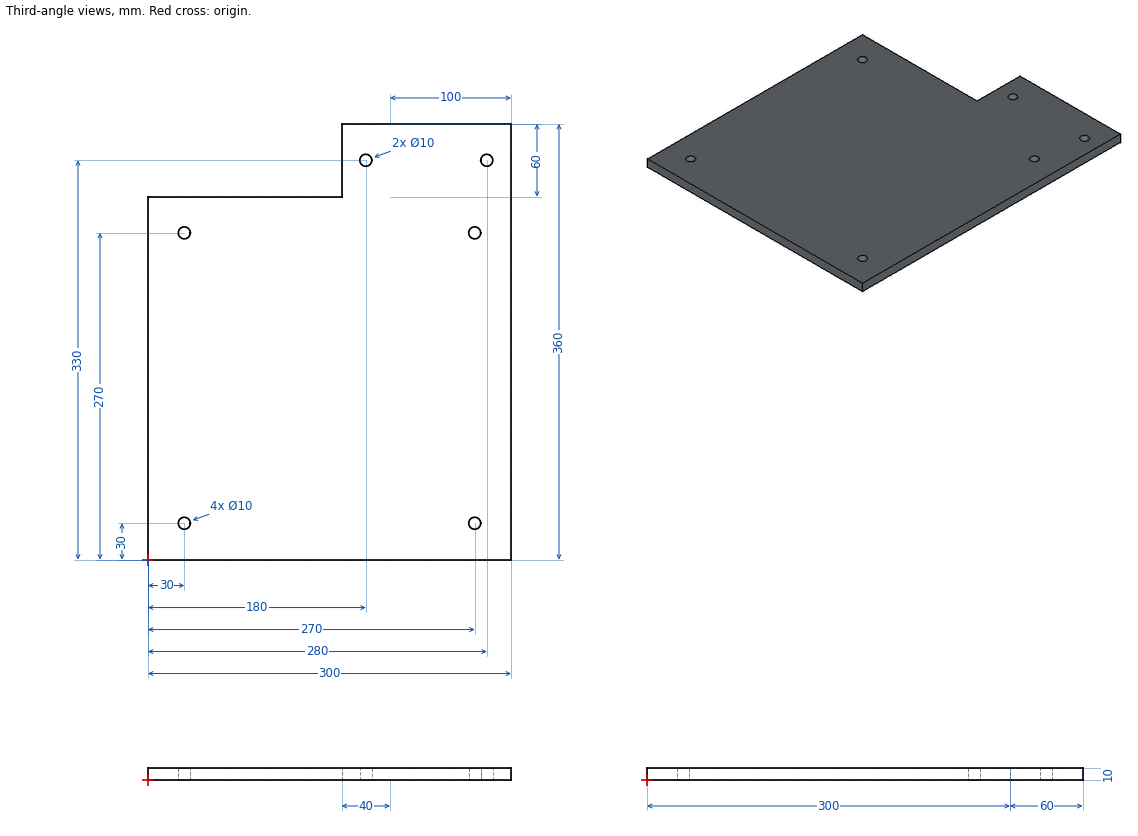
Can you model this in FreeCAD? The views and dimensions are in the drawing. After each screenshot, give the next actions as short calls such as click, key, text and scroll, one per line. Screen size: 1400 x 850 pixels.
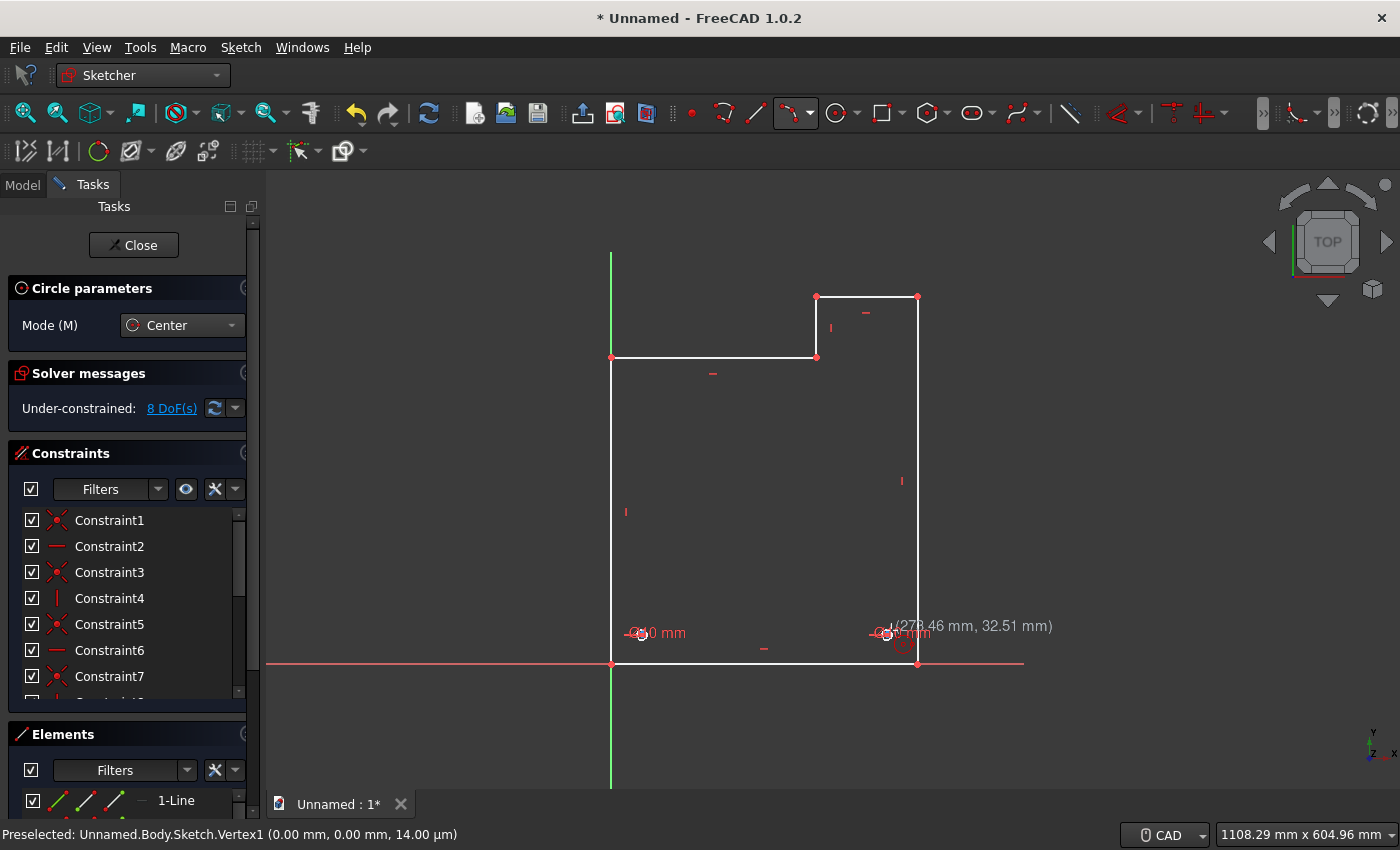
scroll(642, 388, up, 8)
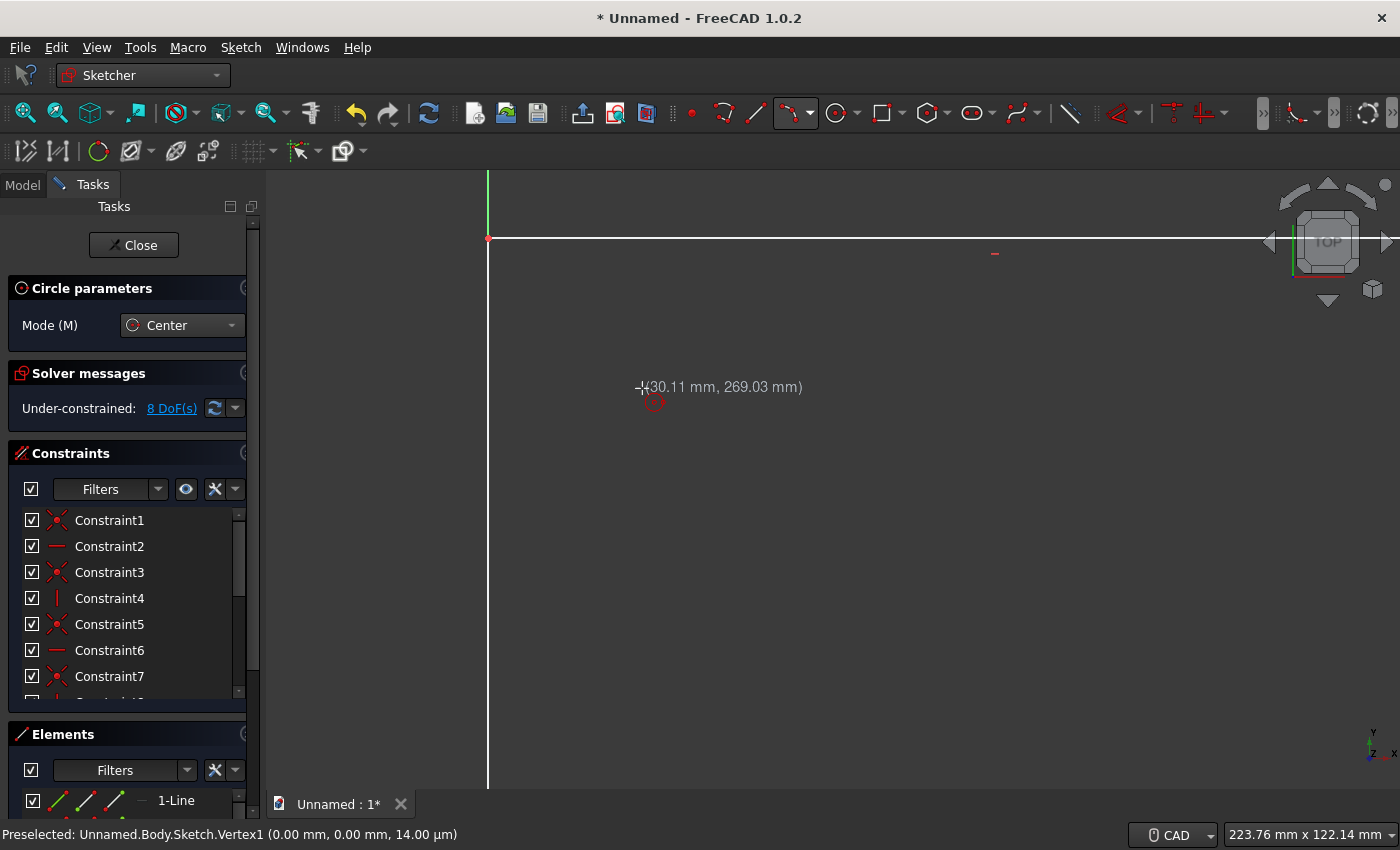
scroll(642, 388, down, 8)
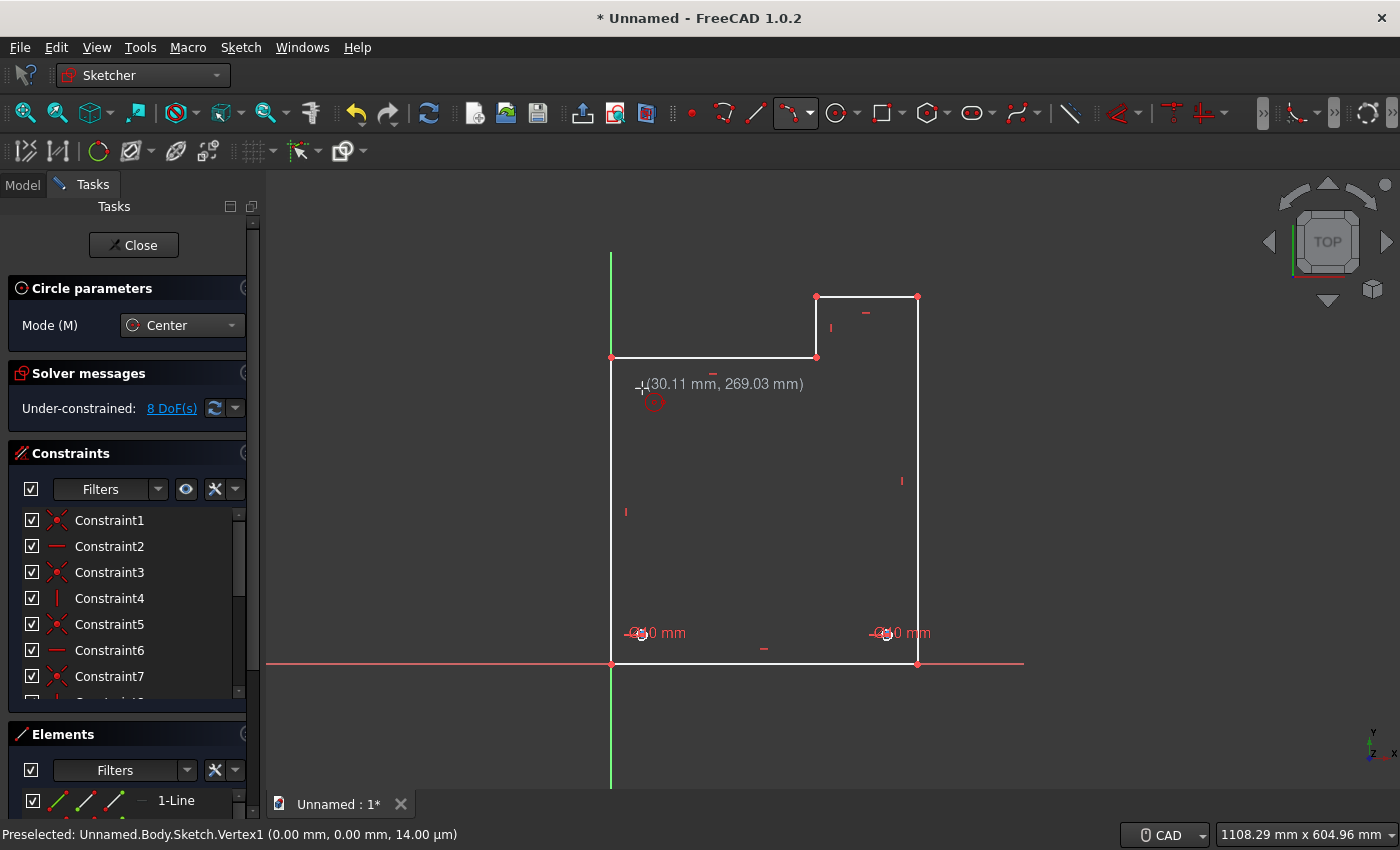
click(642, 388)
move(646, 384)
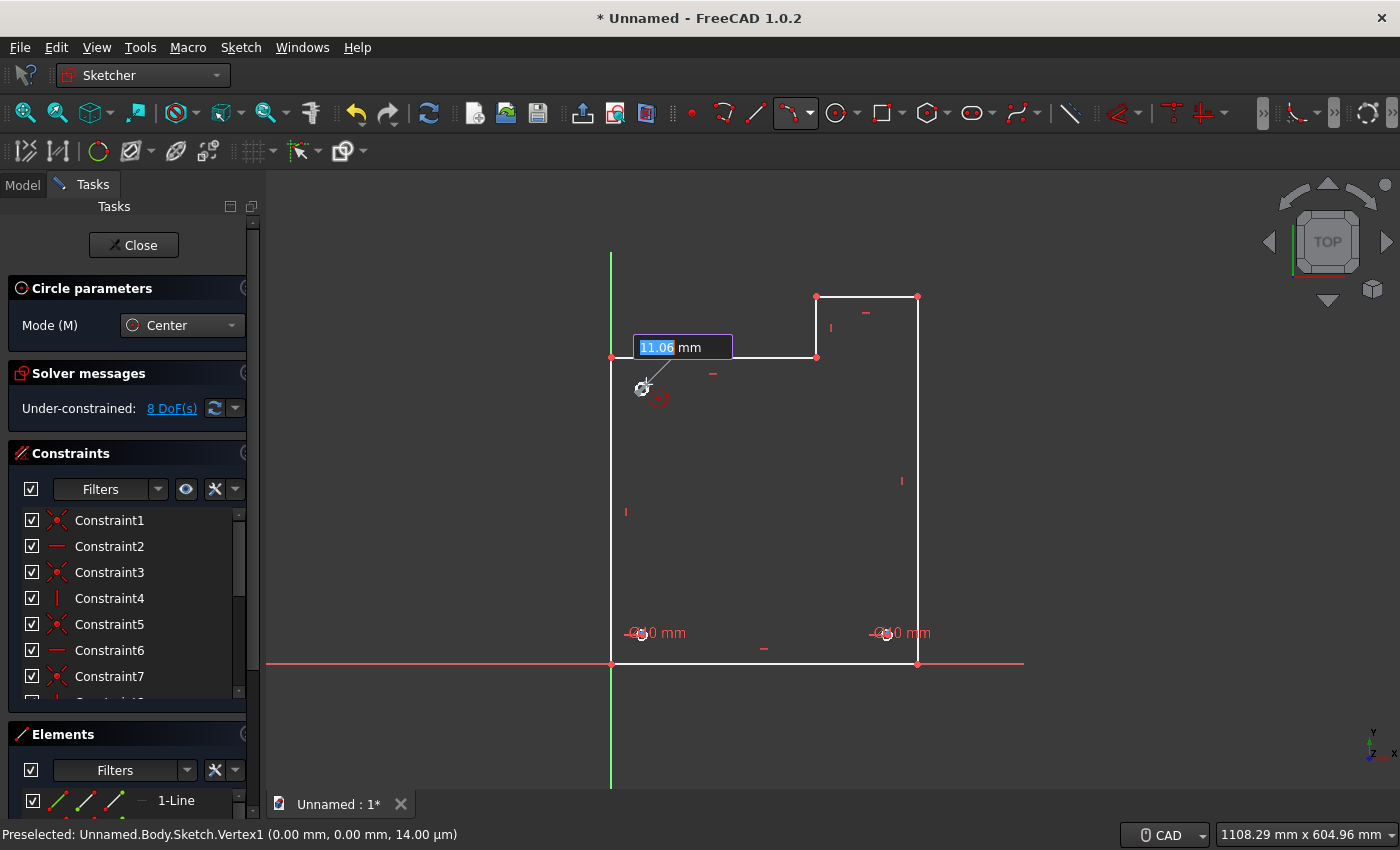
text(10)
key(Return)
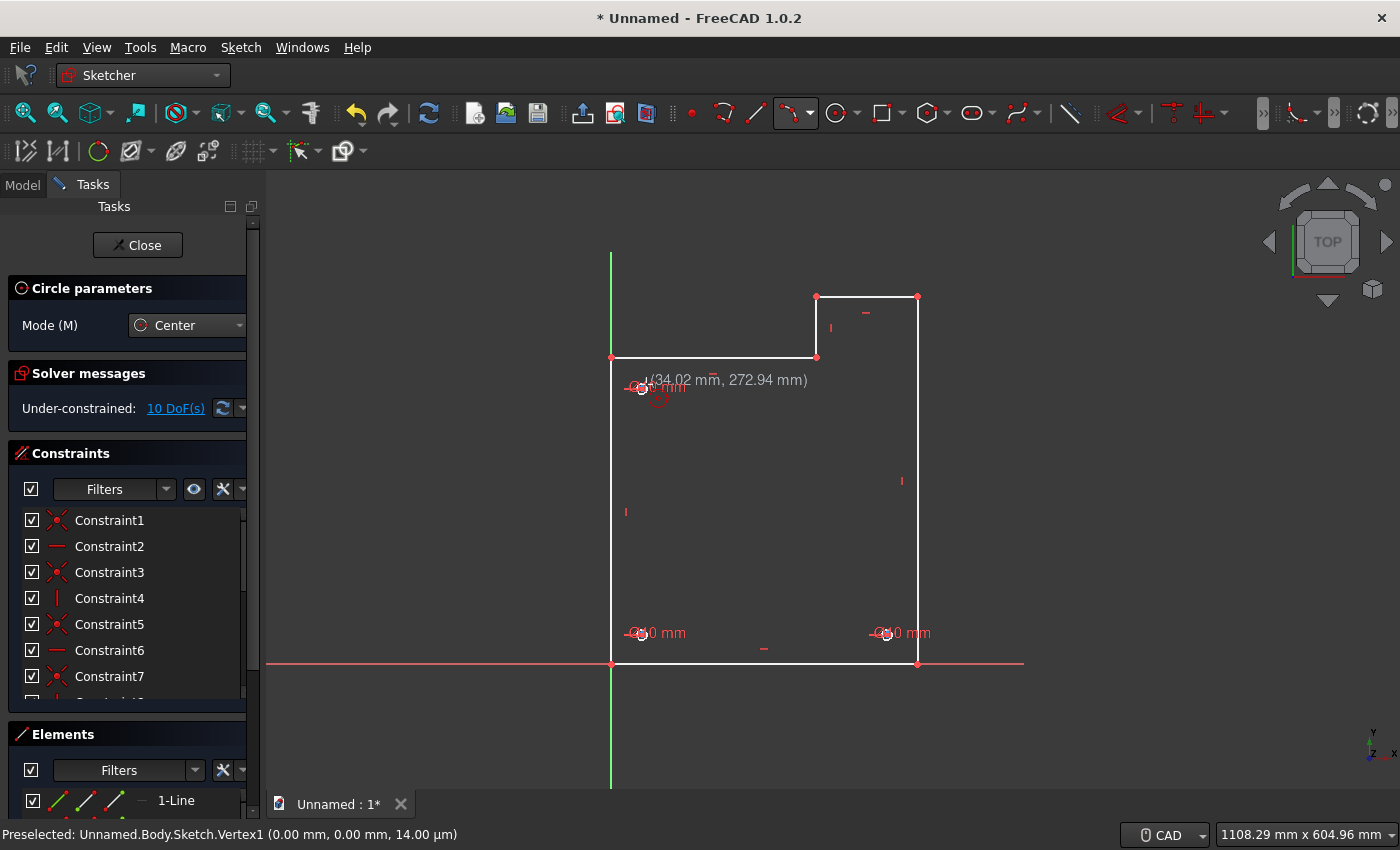
scroll(887, 388, up, 8)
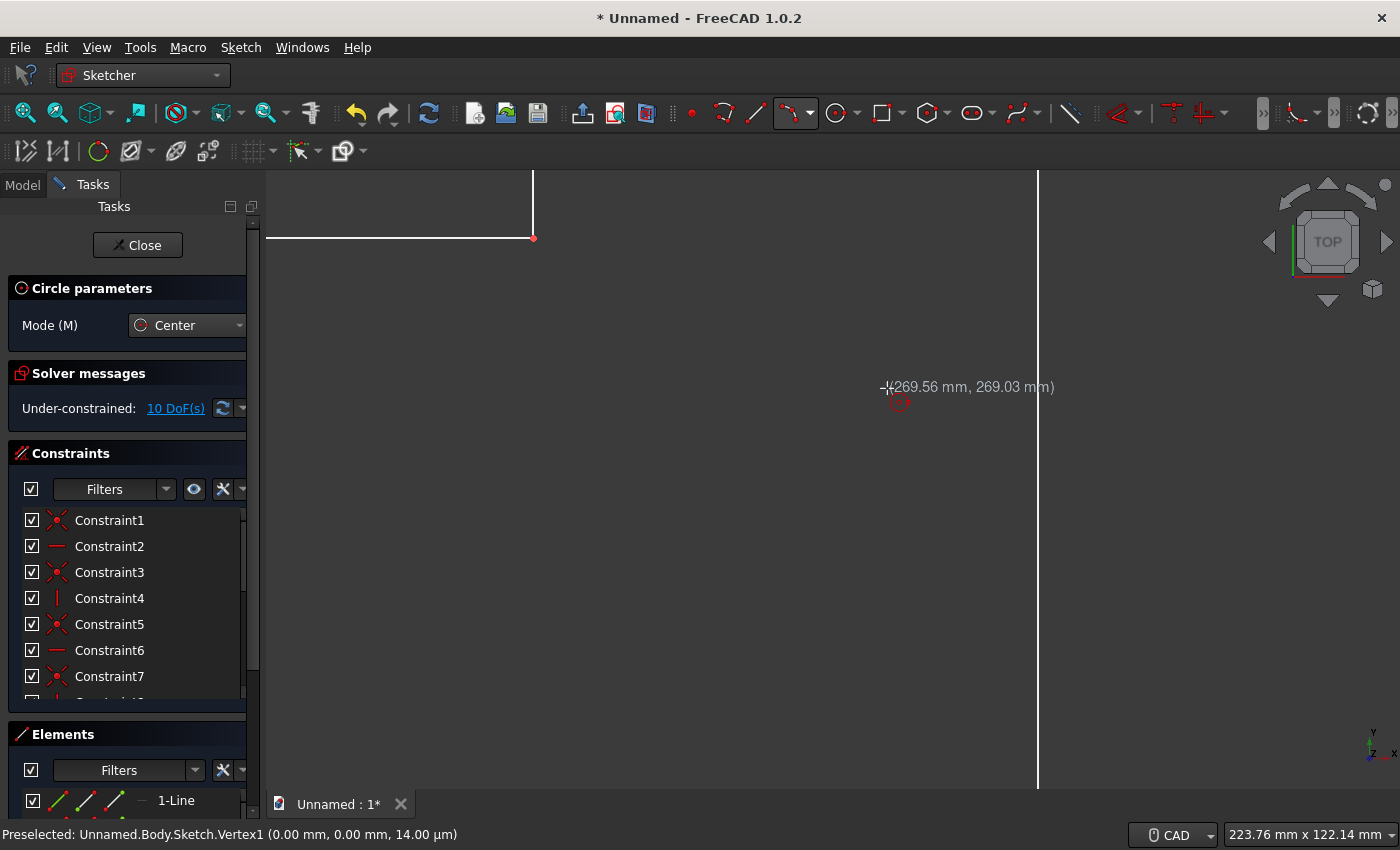
scroll(887, 388, down, 8)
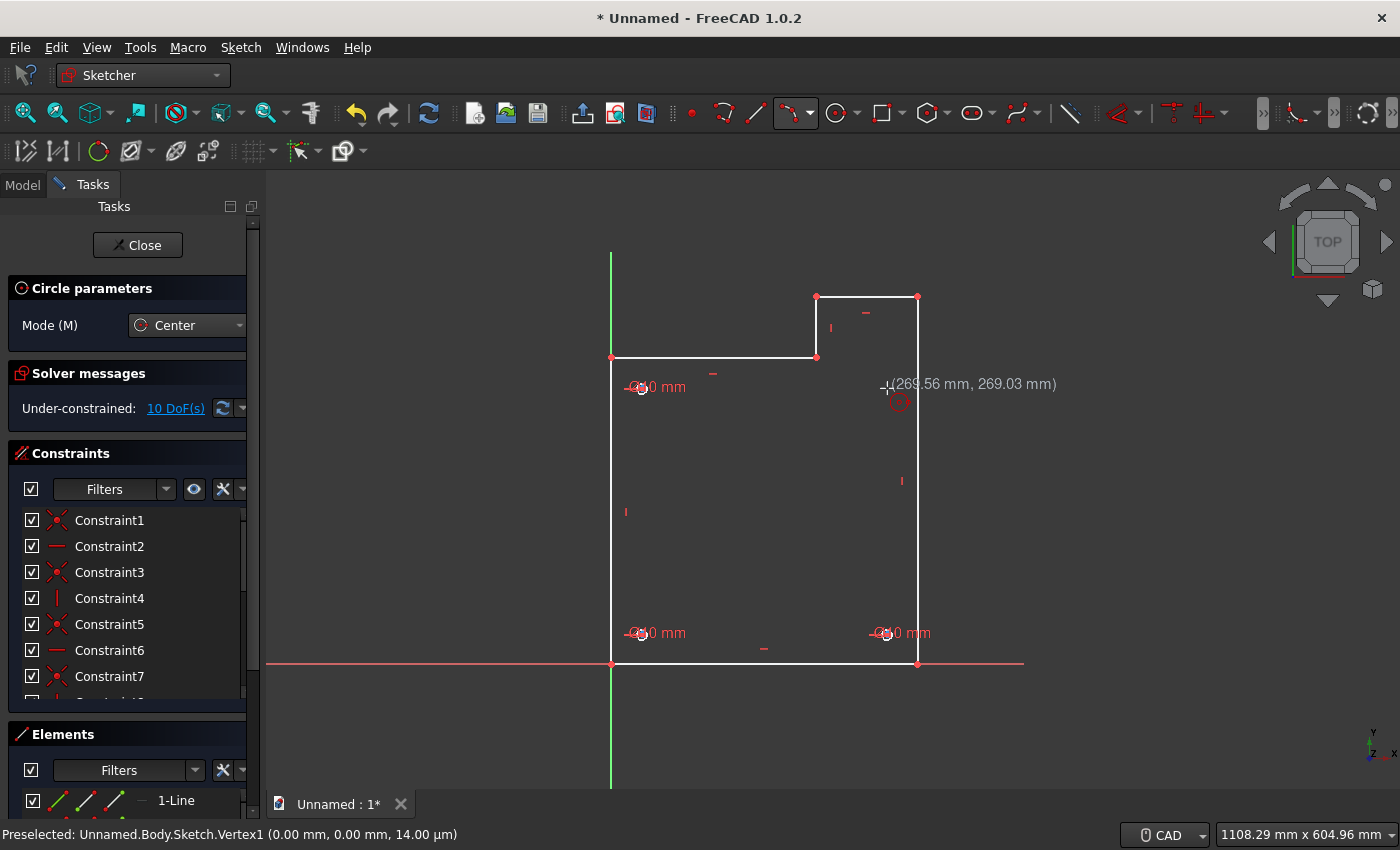
click(887, 388)
move(891, 384)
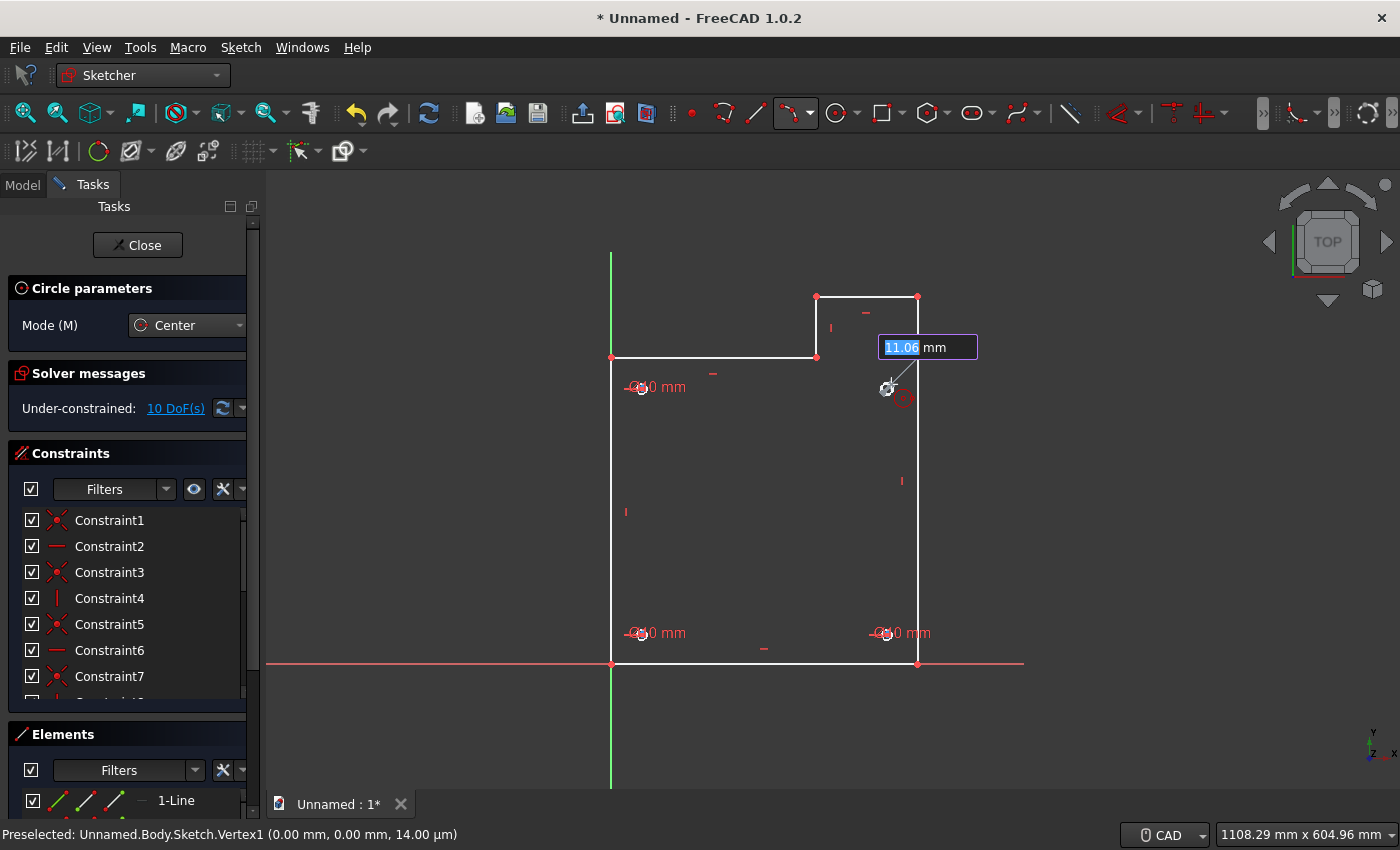
text(10)
key(Return)
key(Escape)